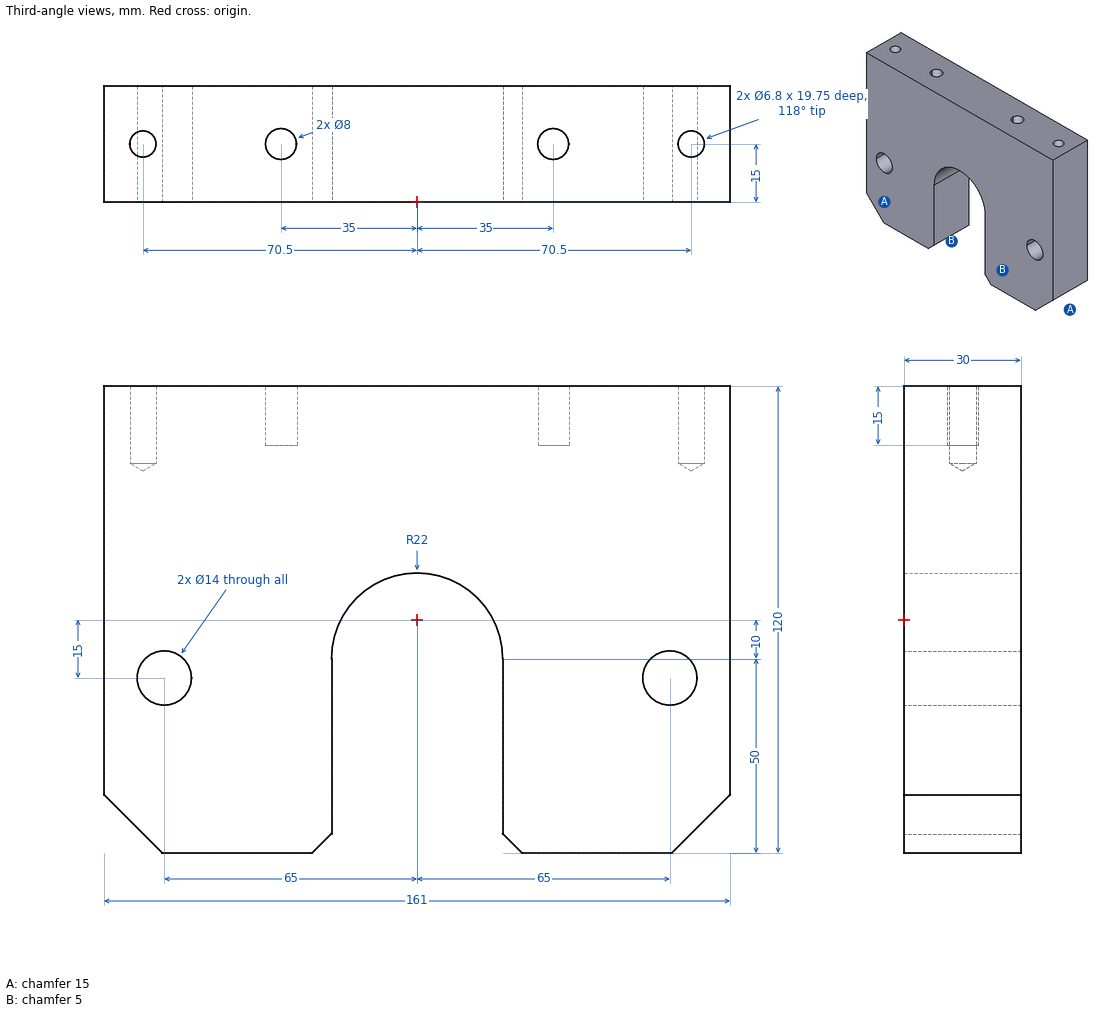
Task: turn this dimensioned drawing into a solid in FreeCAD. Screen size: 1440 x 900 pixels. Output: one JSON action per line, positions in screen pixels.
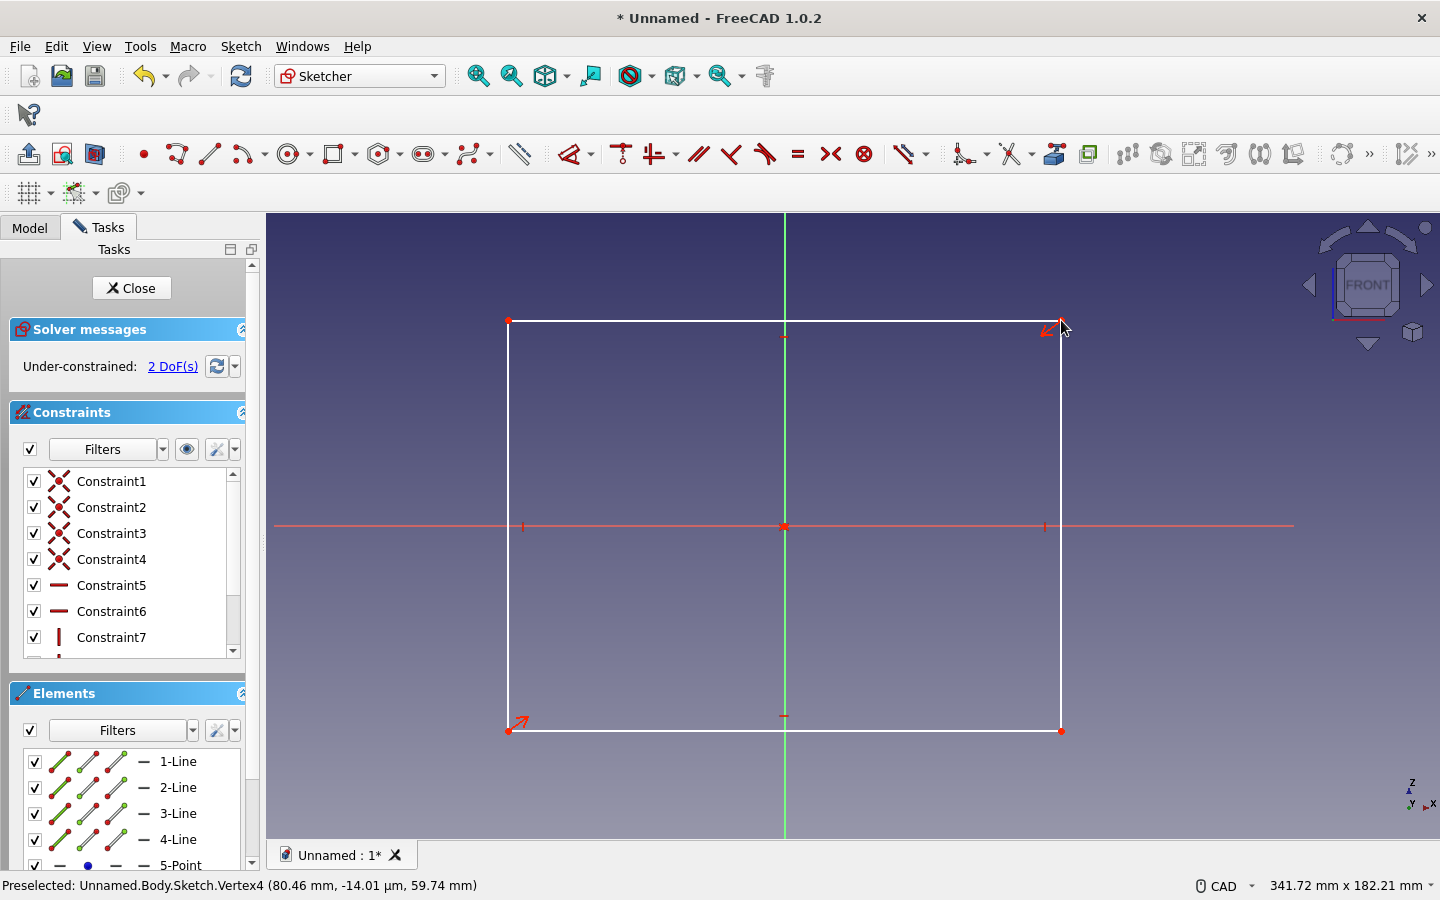
{"action": "left_click", "coordinate": [568, 154]}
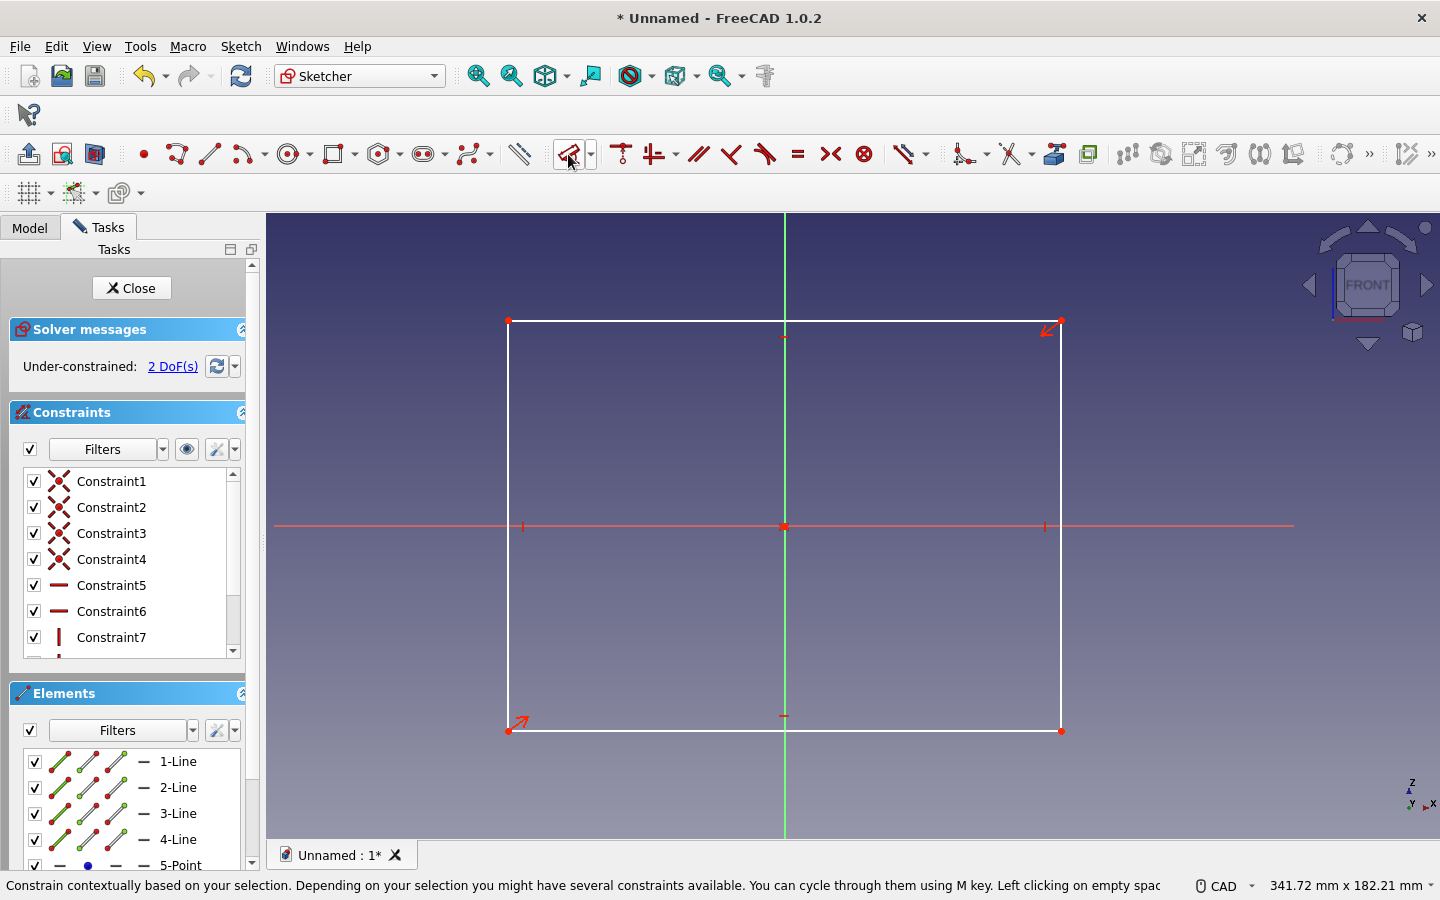
{"action": "left_click", "coordinate": [674, 731]}
{"action": "left_click", "coordinate": [657, 765]}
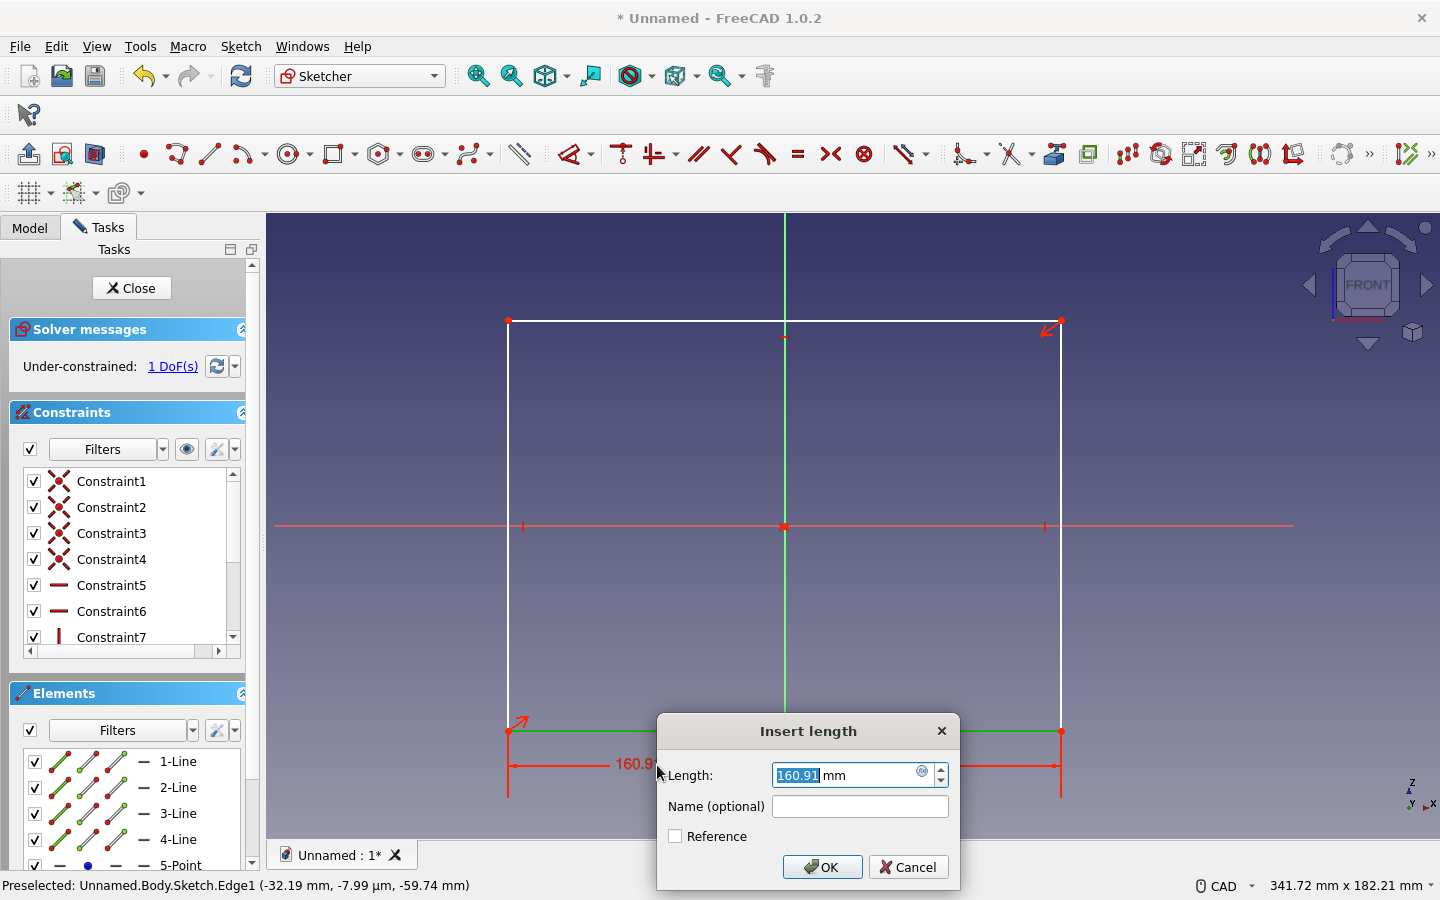
{"action": "type", "text": "161"}
{"action": "key", "text": "Return"}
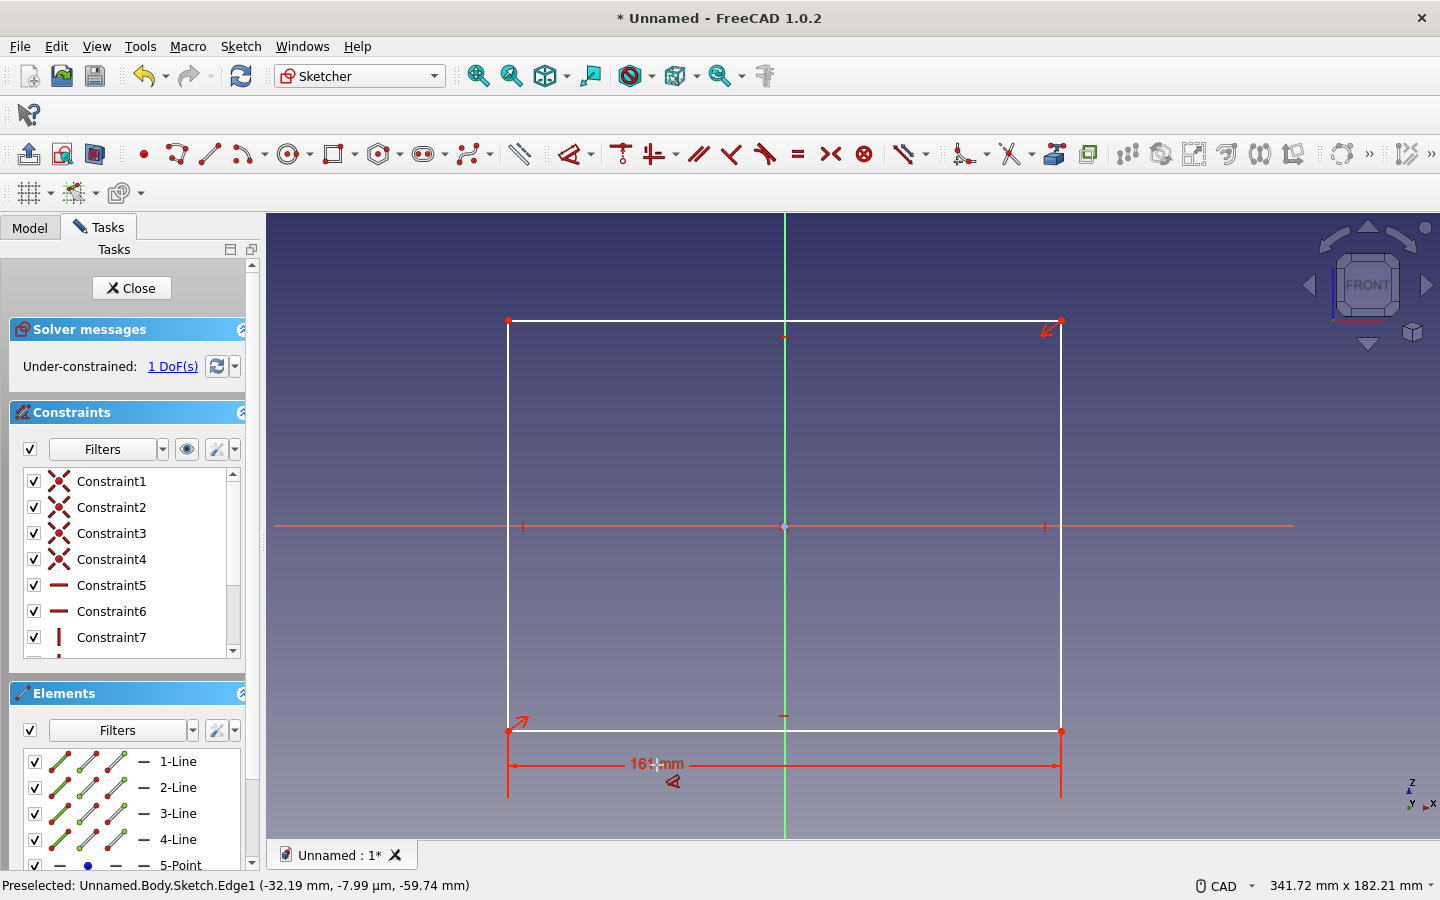
{"action": "left_click", "coordinate": [1061, 608]}
{"action": "left_click", "coordinate": [1095, 432]}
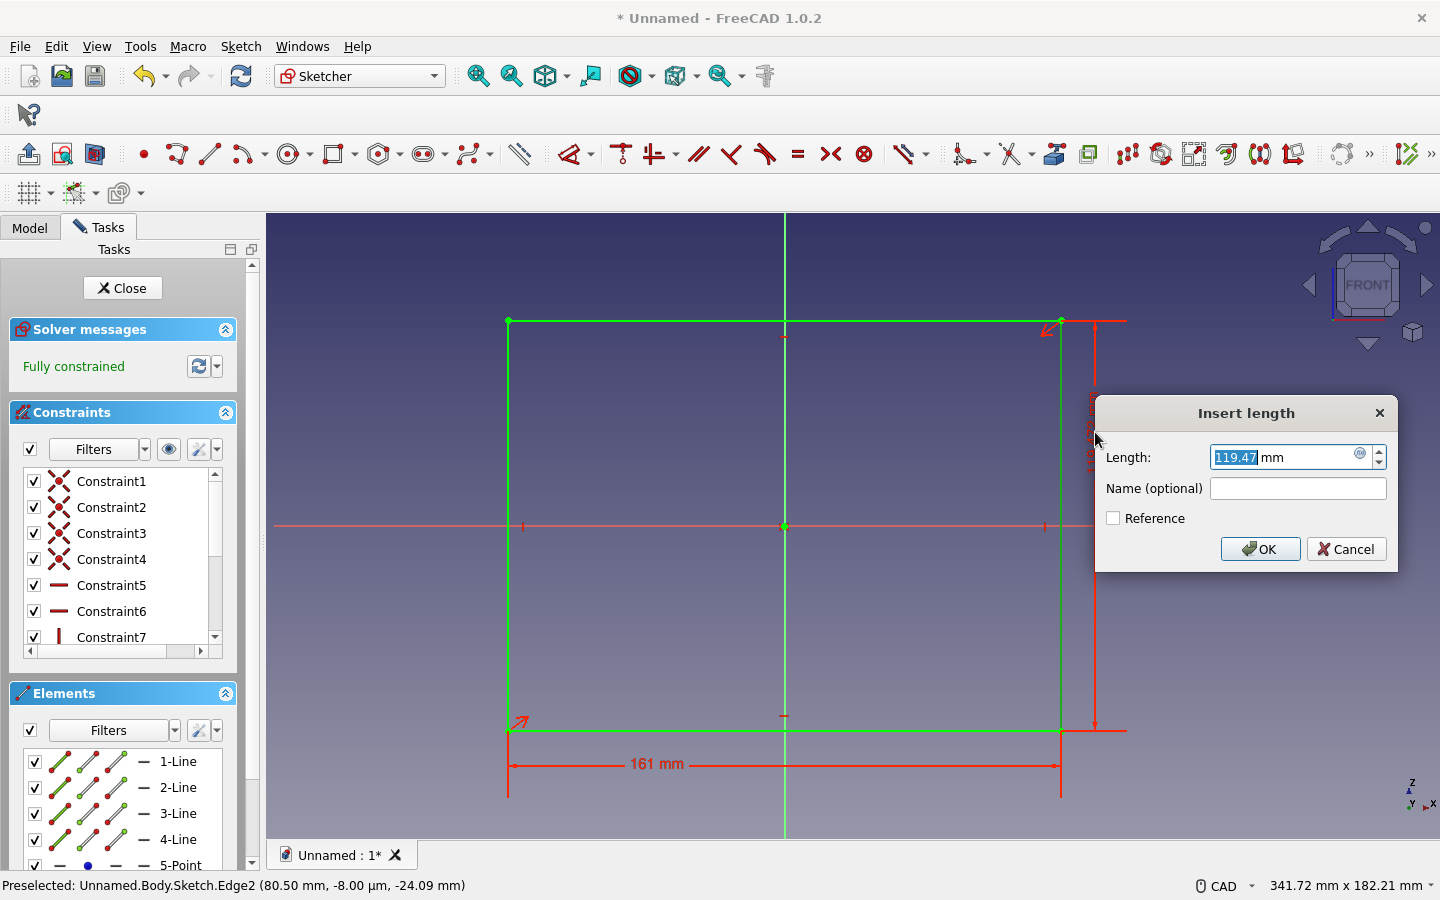
{"action": "type", "text": "120"}
{"action": "key", "text": "Return"}
{"action": "key", "text": "Escape"}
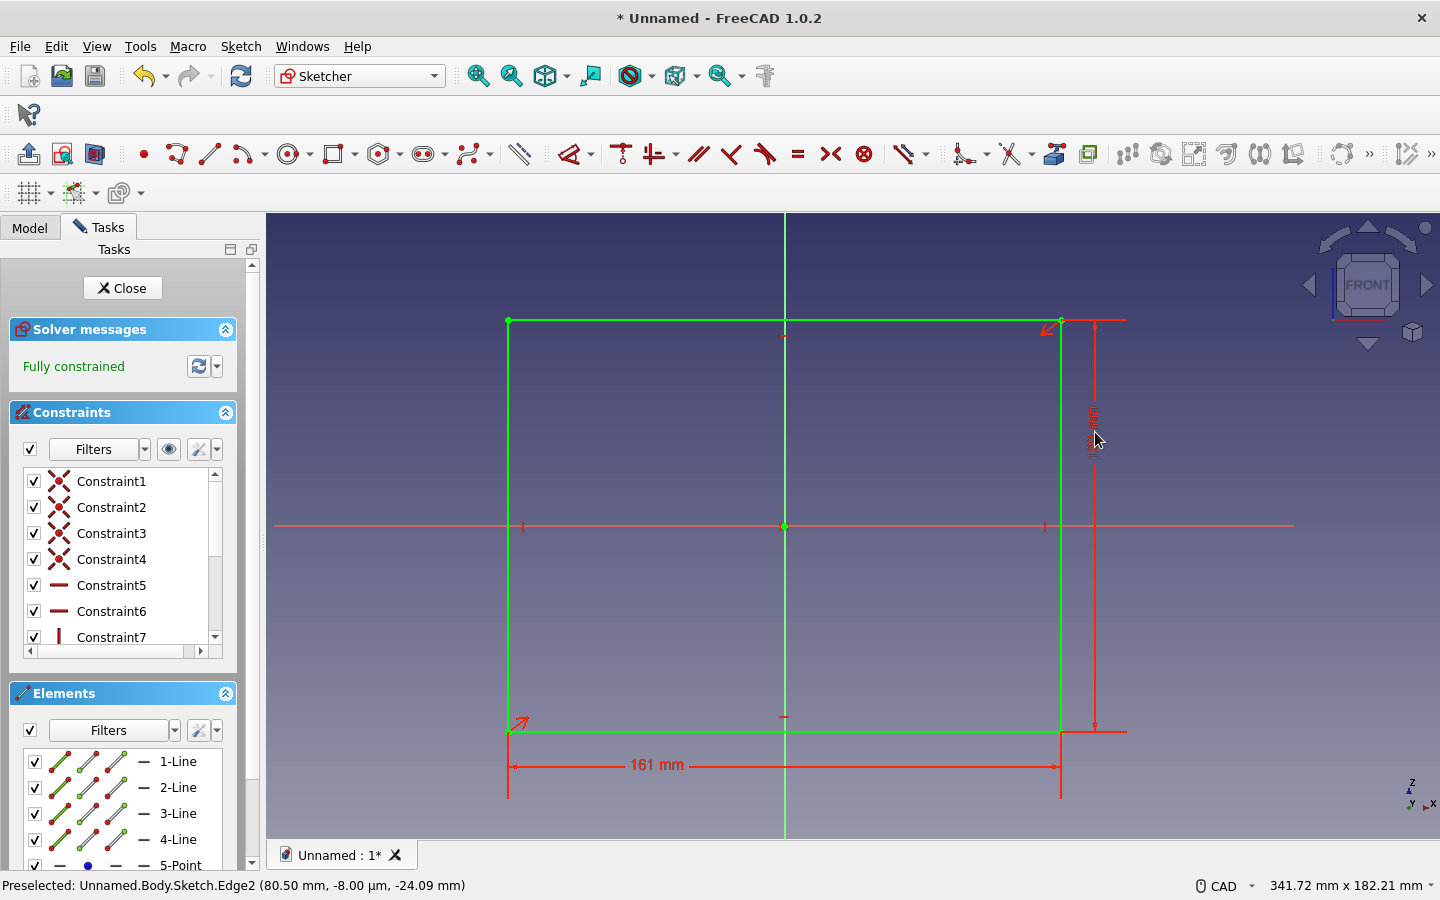
{"action": "left_click", "coordinate": [123, 288]}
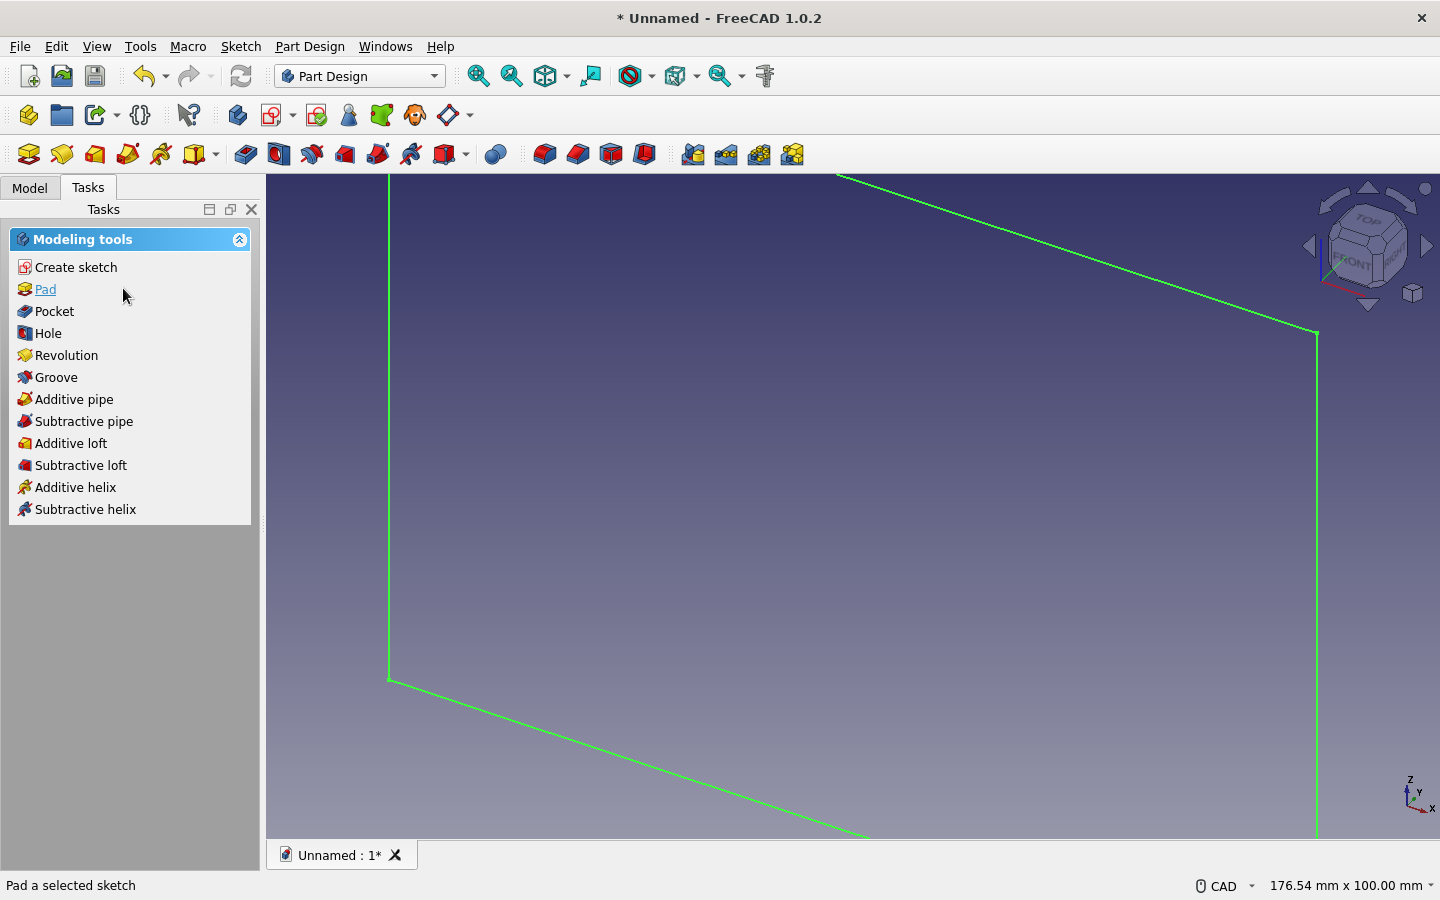
{"action": "left_click", "coordinate": [29, 154]}